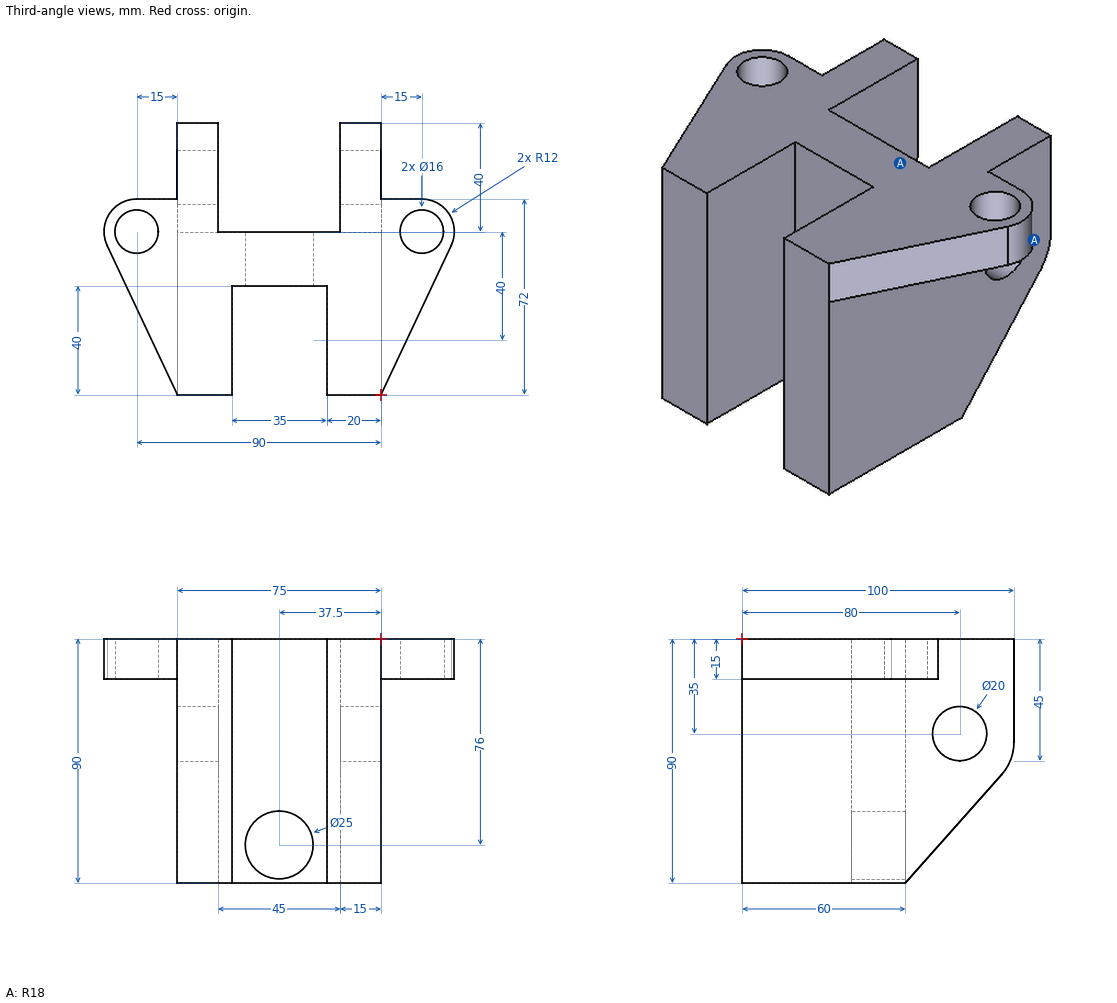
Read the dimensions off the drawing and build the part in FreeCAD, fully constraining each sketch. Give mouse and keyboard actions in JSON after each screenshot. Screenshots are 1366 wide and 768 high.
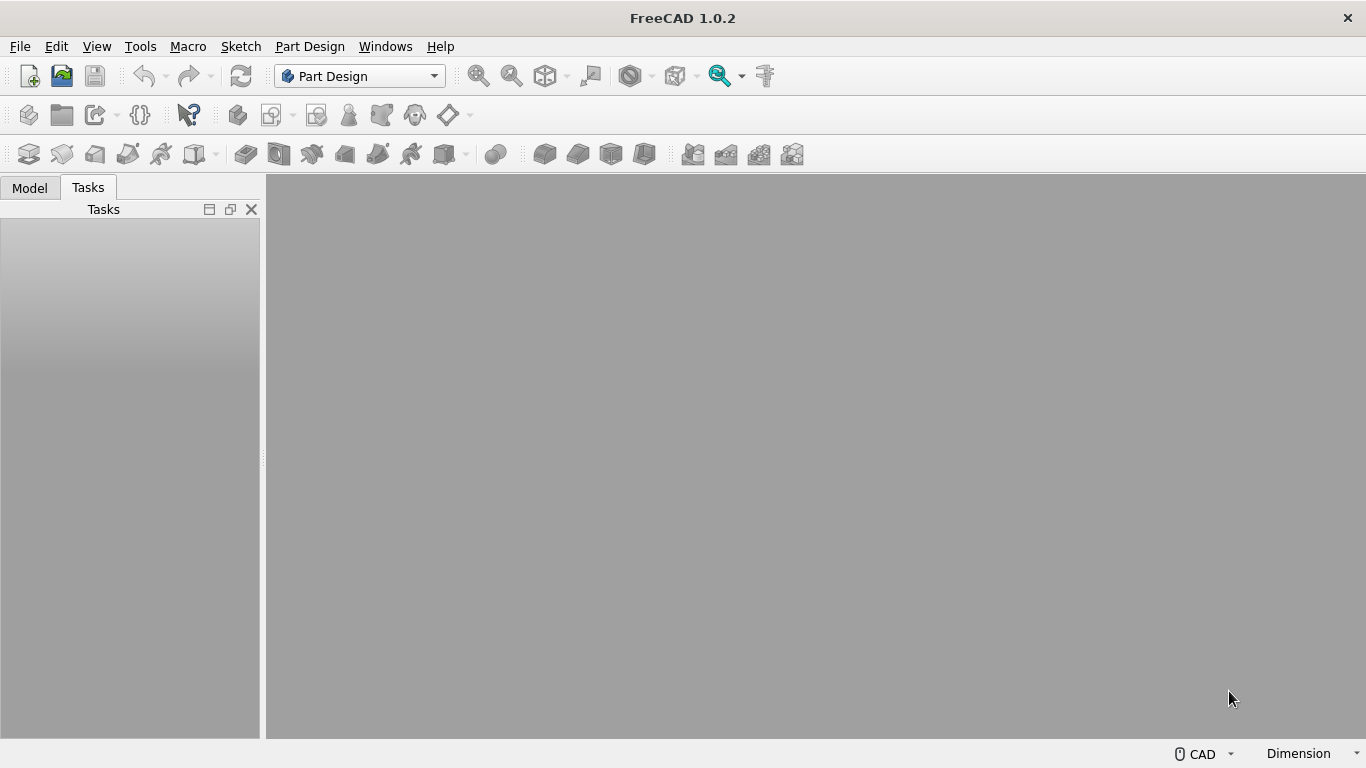
{"action": "key", "text": "ctrl+n"}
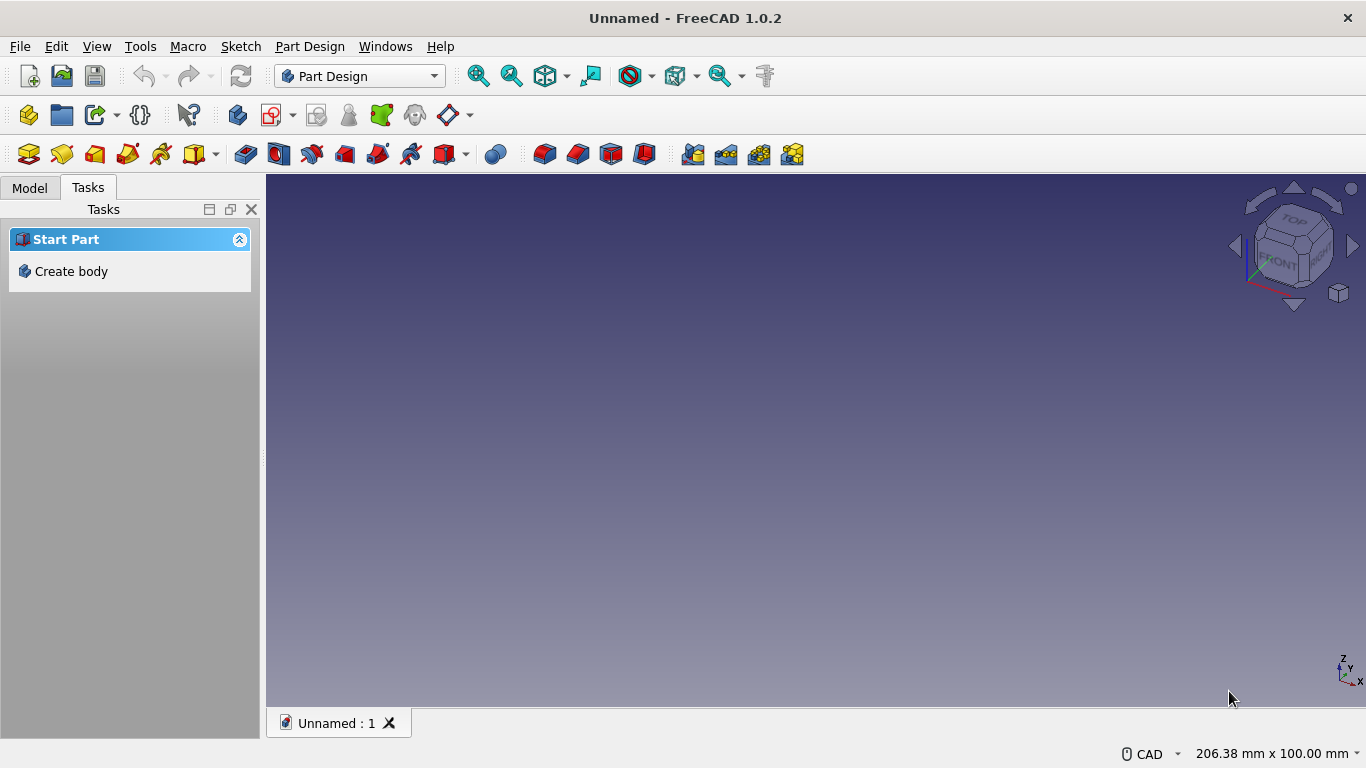
{"action": "left_click", "coordinate": [270, 116]}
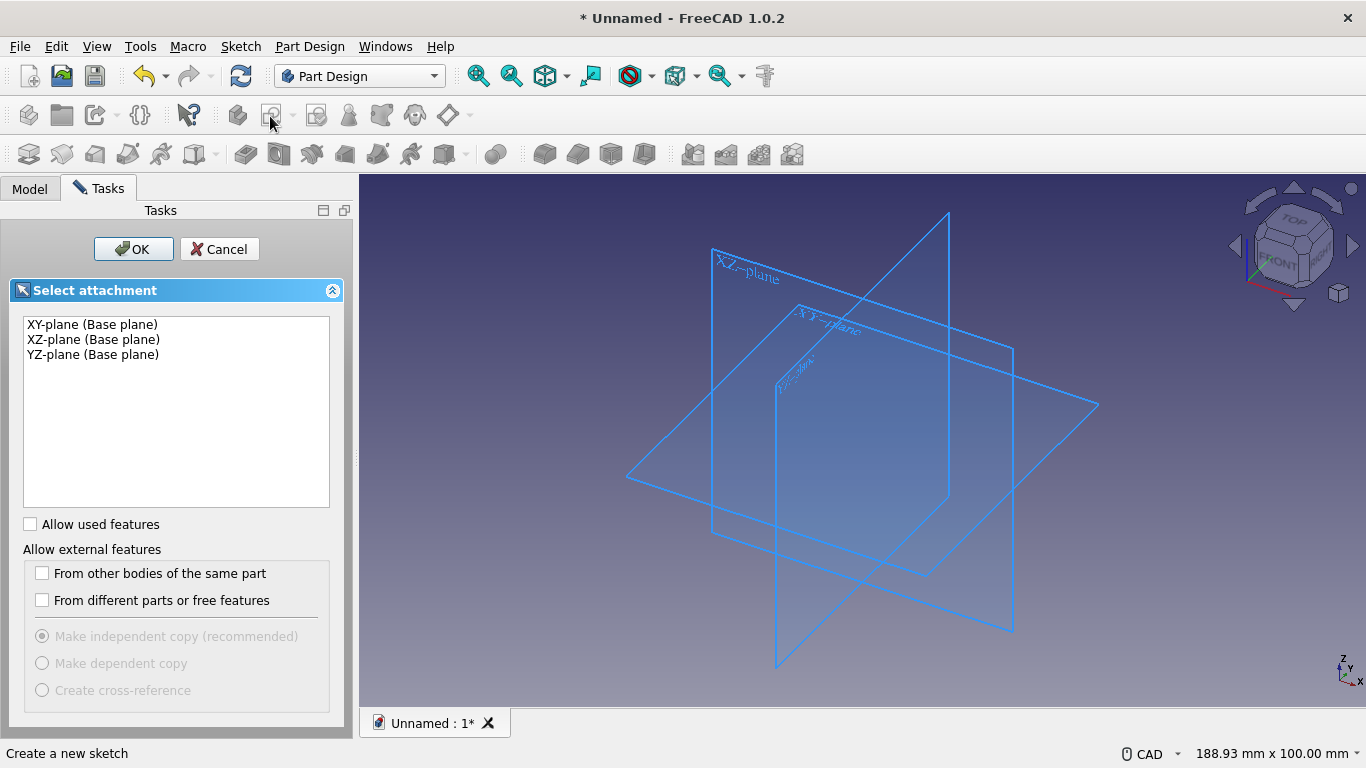
{"action": "left_click", "coordinate": [84, 354]}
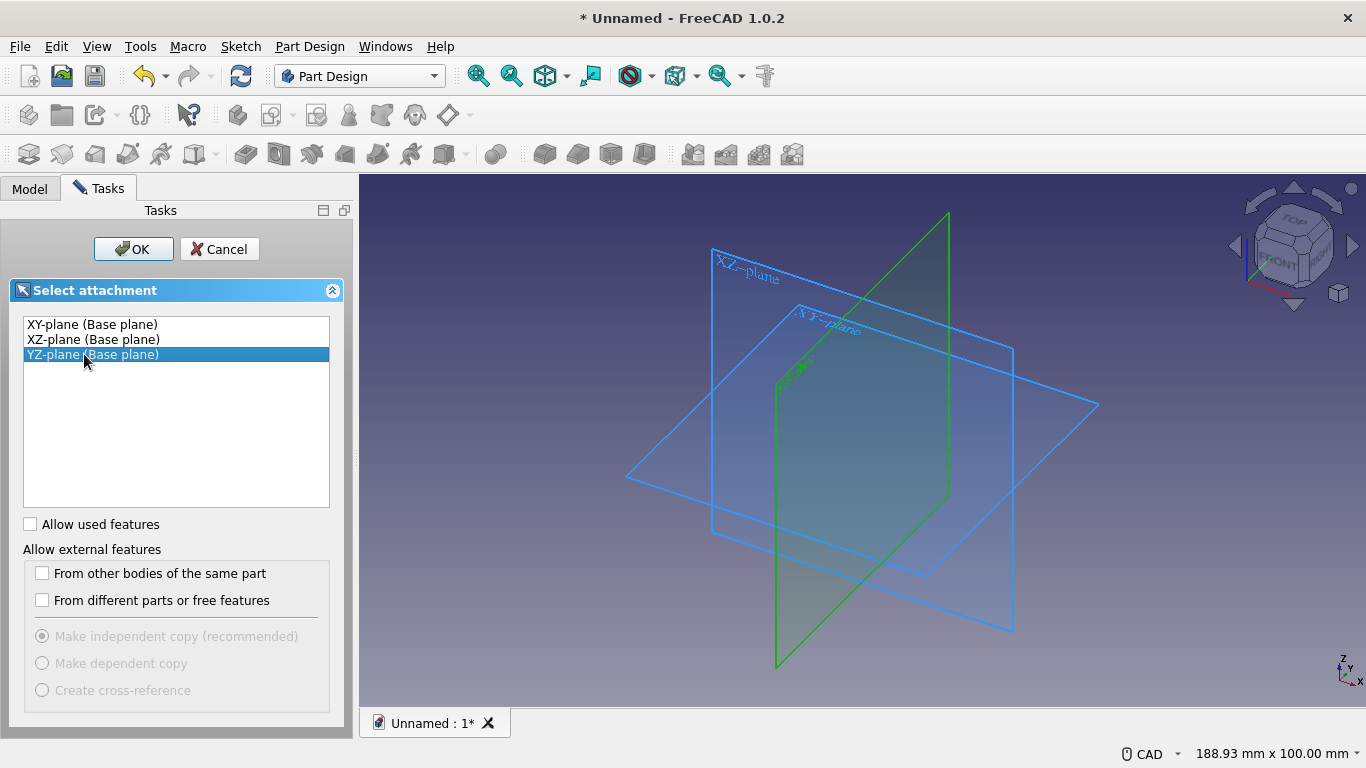
{"action": "left_click", "coordinate": [134, 249]}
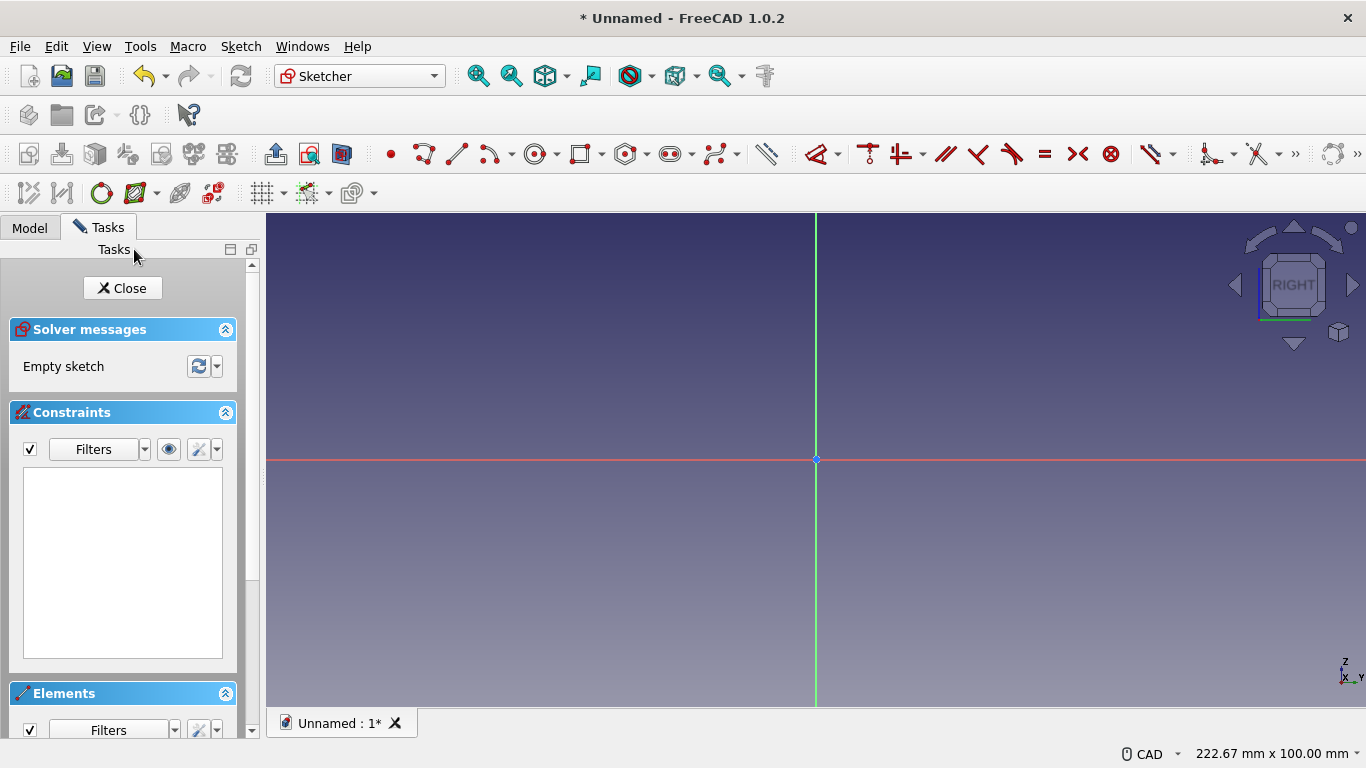
{"action": "scroll", "coordinate": [364, 241], "scroll_direction": "down", "scroll_amount": 3}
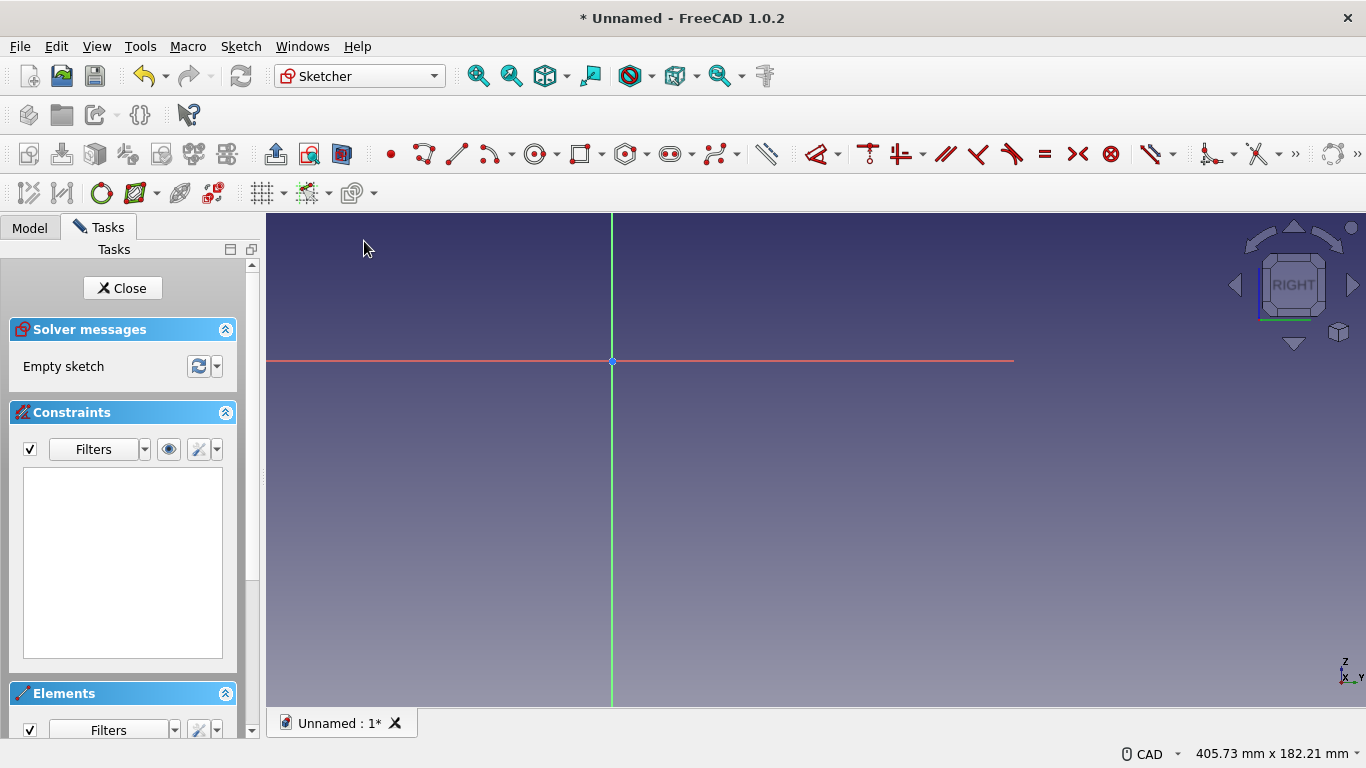
{"action": "left_click", "coordinate": [424, 154]}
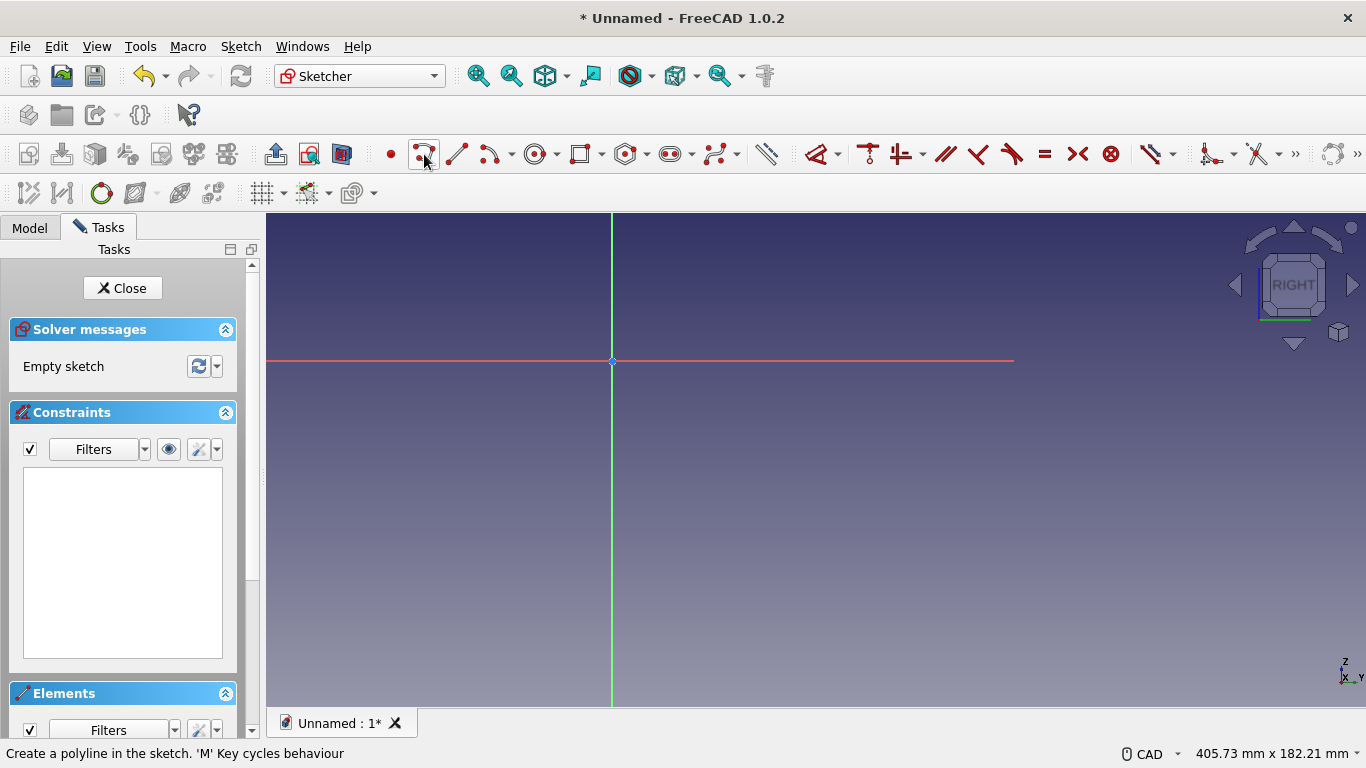
{"action": "left_click", "coordinate": [612, 361]}
{"action": "left_click", "coordinate": [621, 605]}
{"action": "left_click", "coordinate": [775, 605]}
{"action": "left_click", "coordinate": [883, 483]}
{"action": "left_click", "coordinate": [883, 370]}
{"action": "left_click", "coordinate": [612, 361]}
{"action": "key", "text": "Escape"}
{"action": "key", "text": "Escape"}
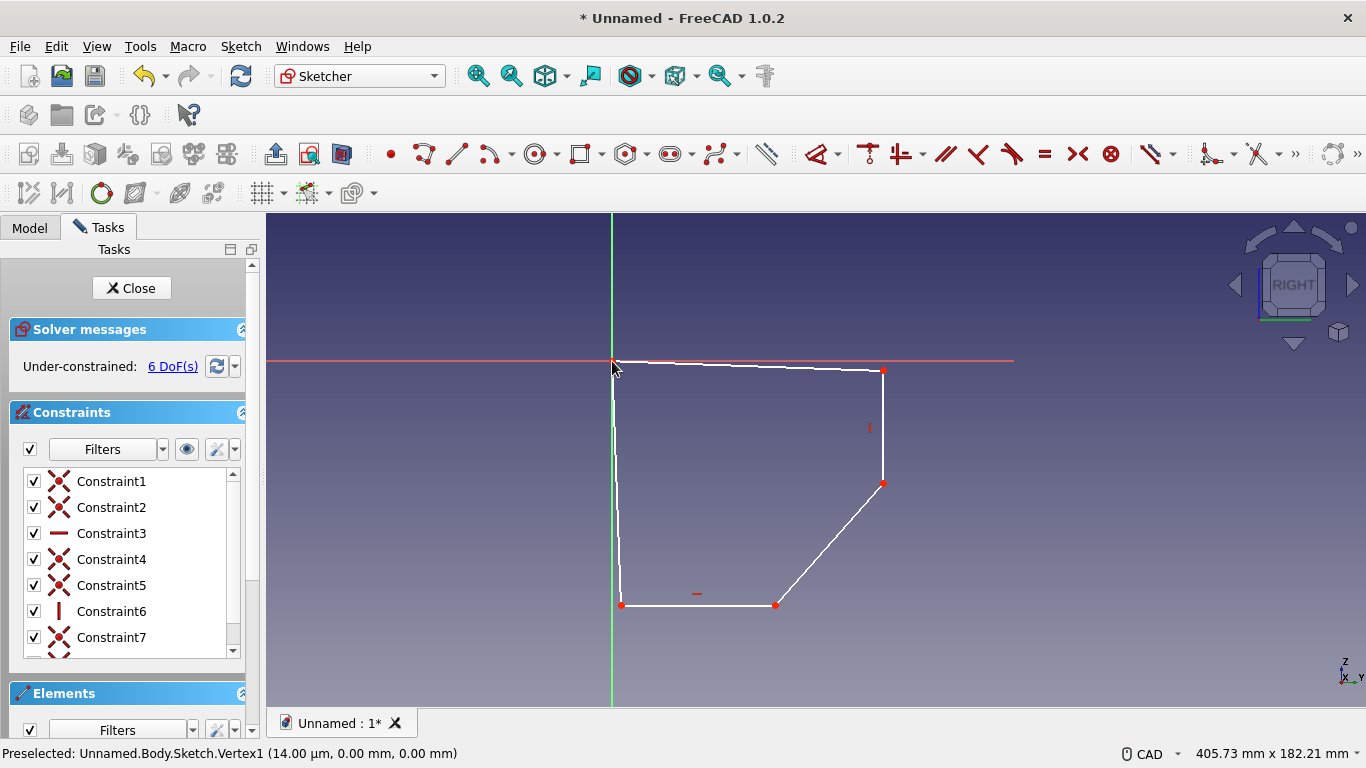
{"action": "left_click", "coordinate": [615, 435]}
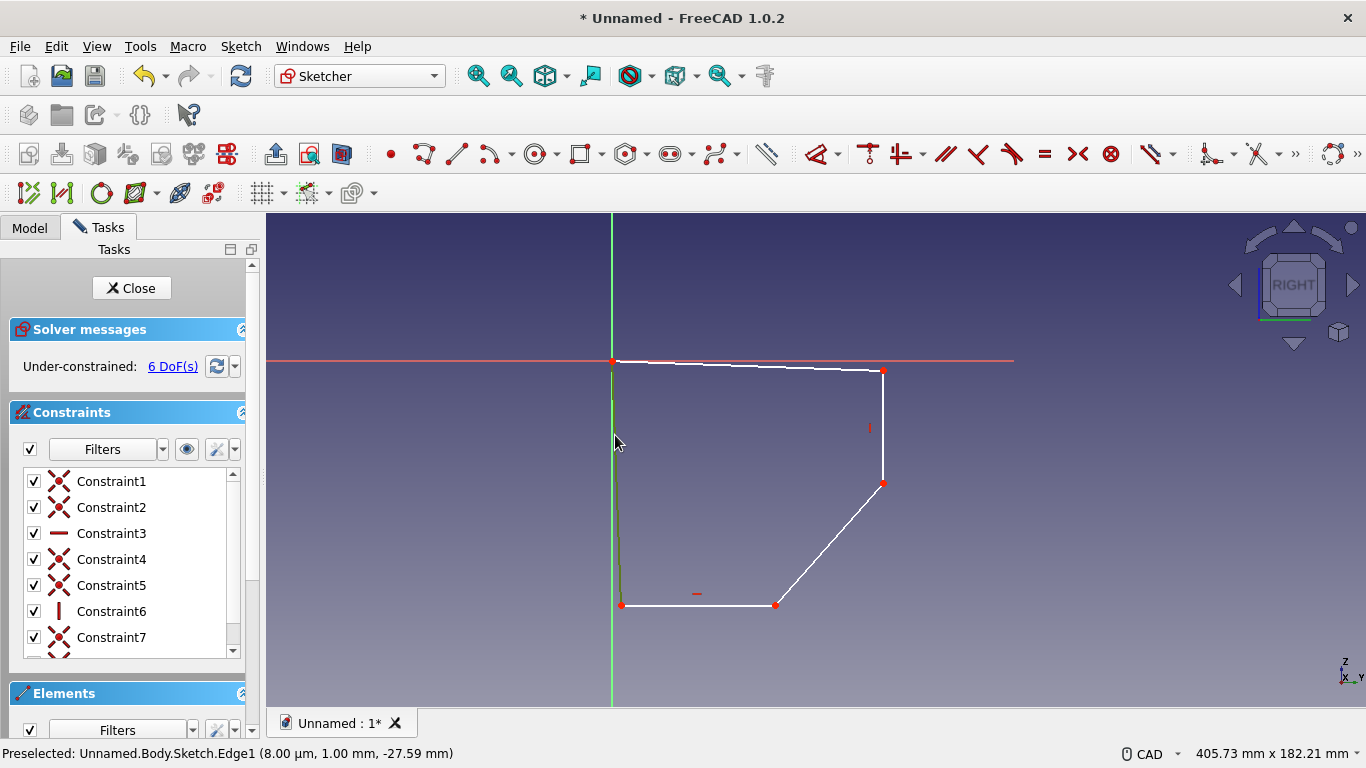
{"action": "left_click", "coordinate": [922, 154]}